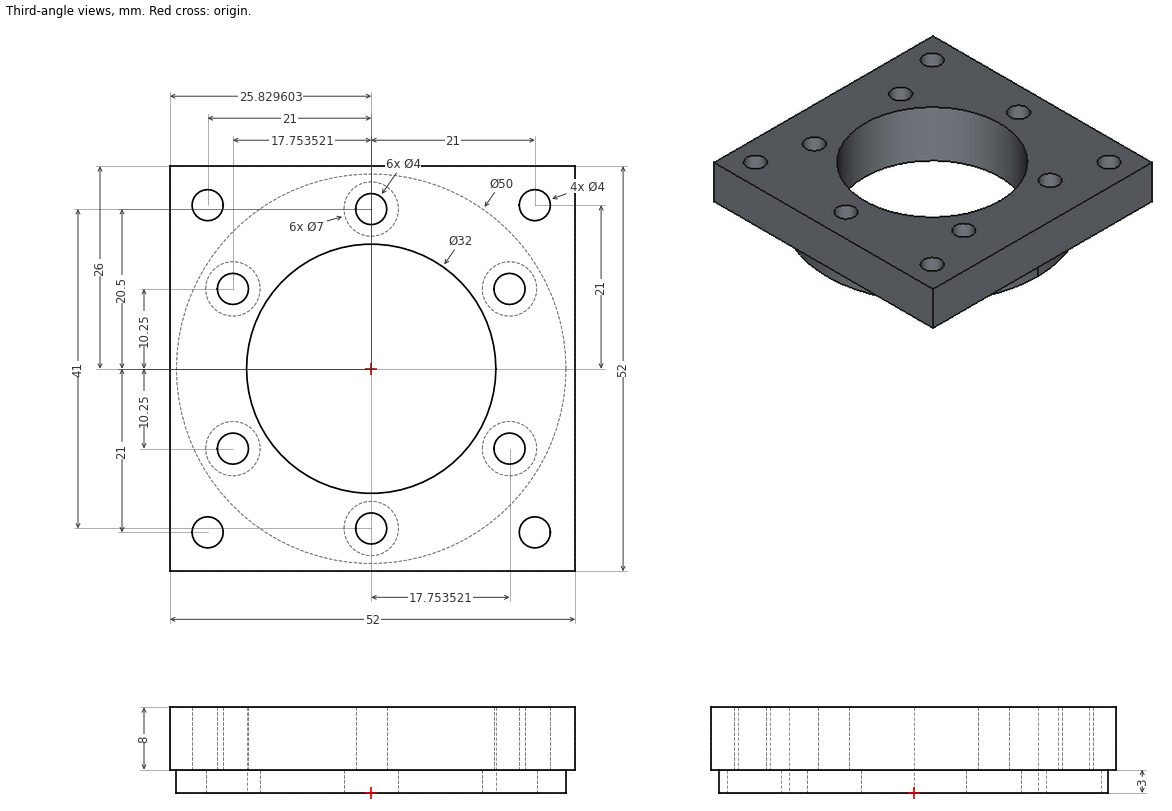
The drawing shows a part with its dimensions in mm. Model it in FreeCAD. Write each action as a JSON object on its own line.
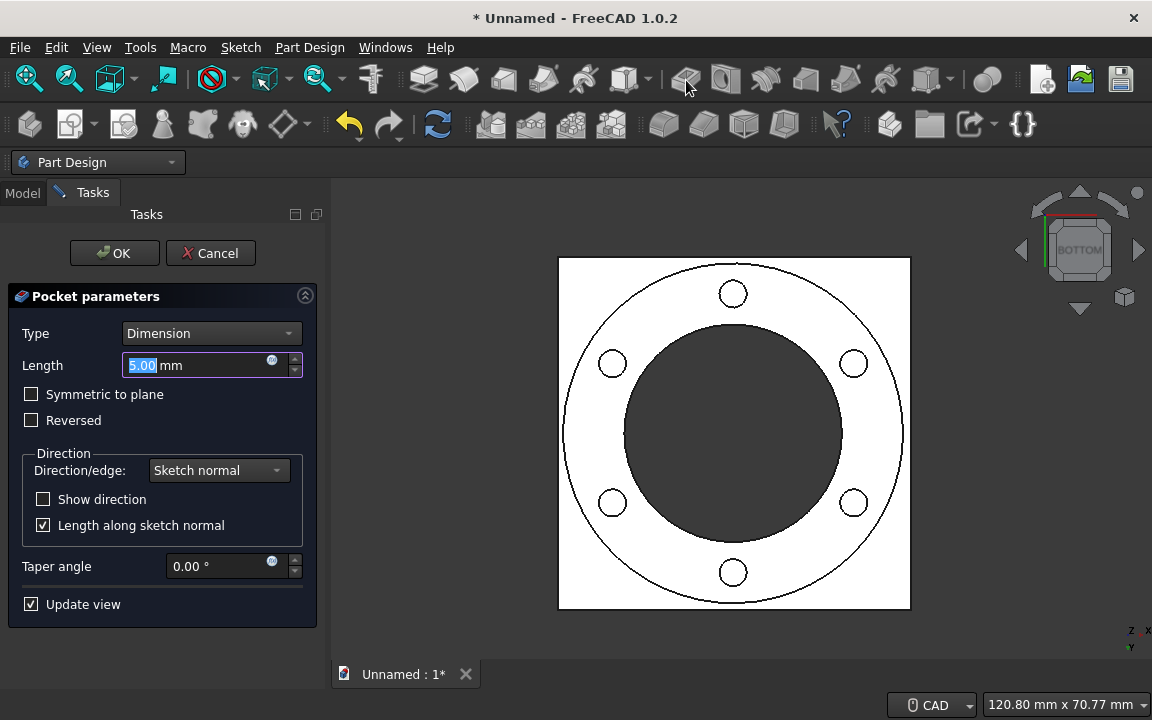
{"action": "left_click", "coordinate": [212, 334]}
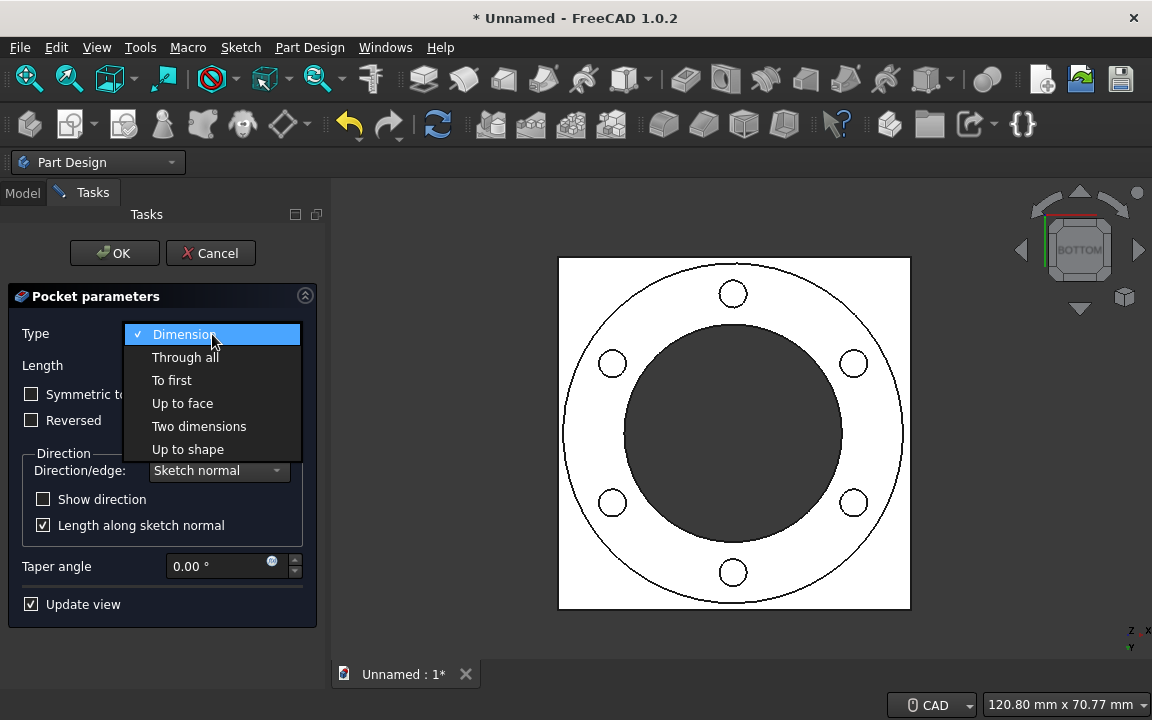
{"action": "left_click", "coordinate": [212, 358]}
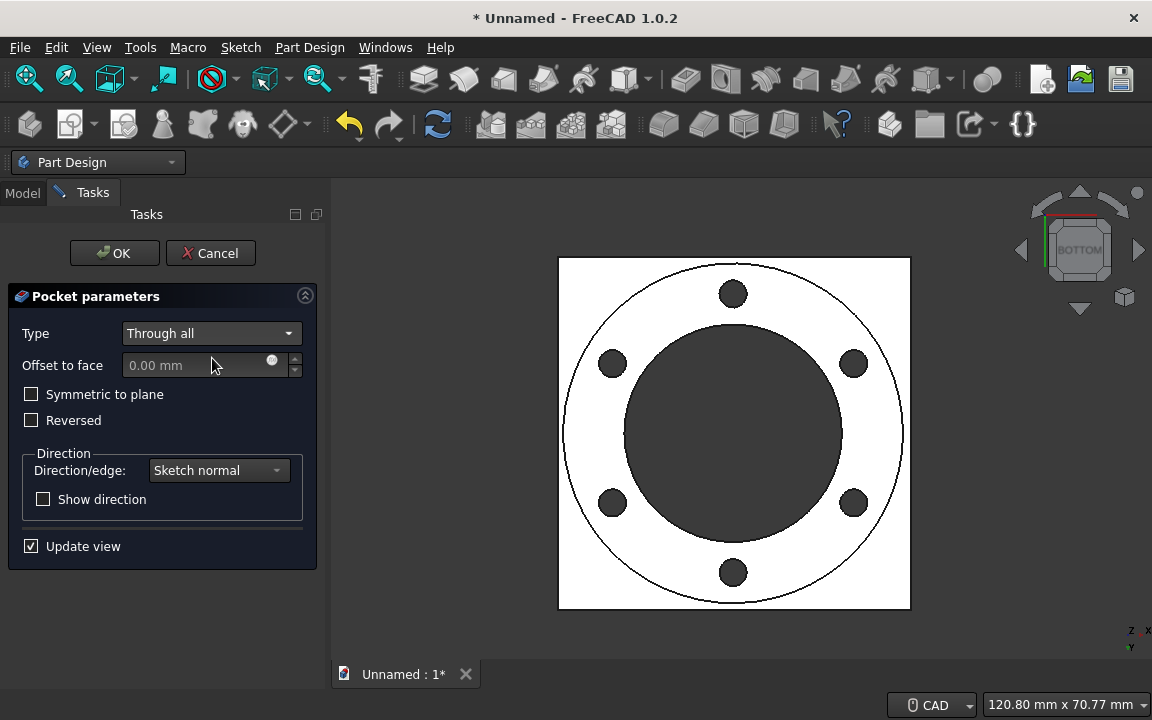
{"action": "left_click", "coordinate": [115, 253]}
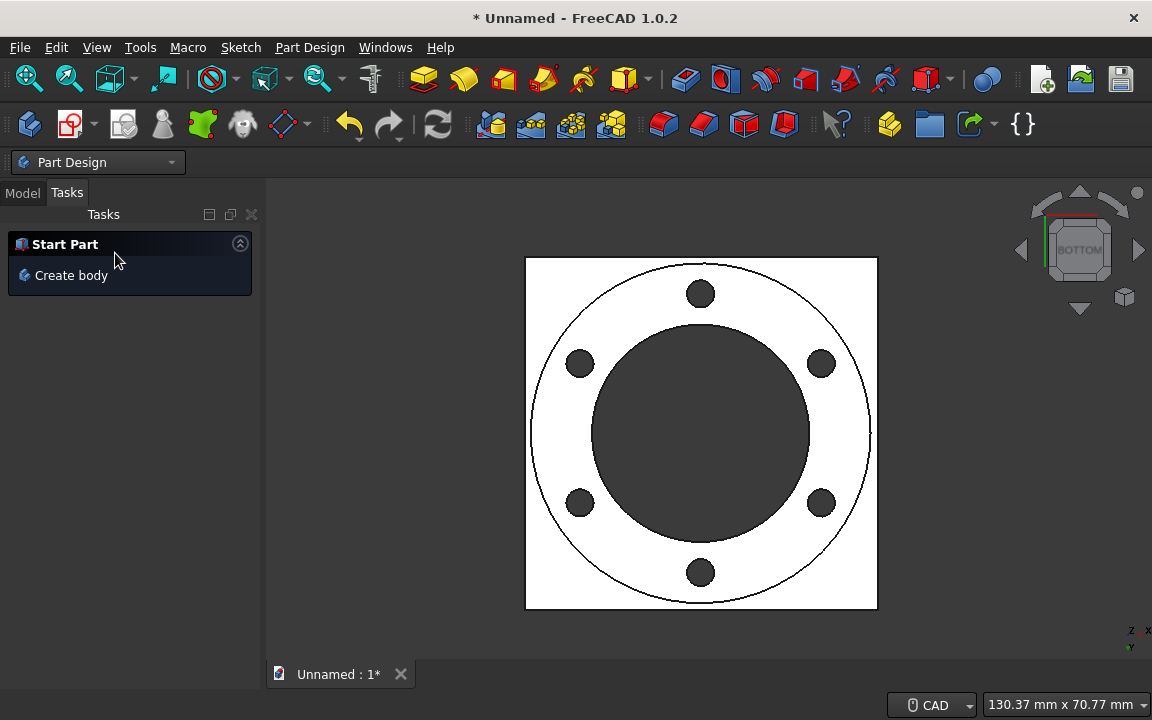
{"action": "left_click", "coordinate": [853, 584]}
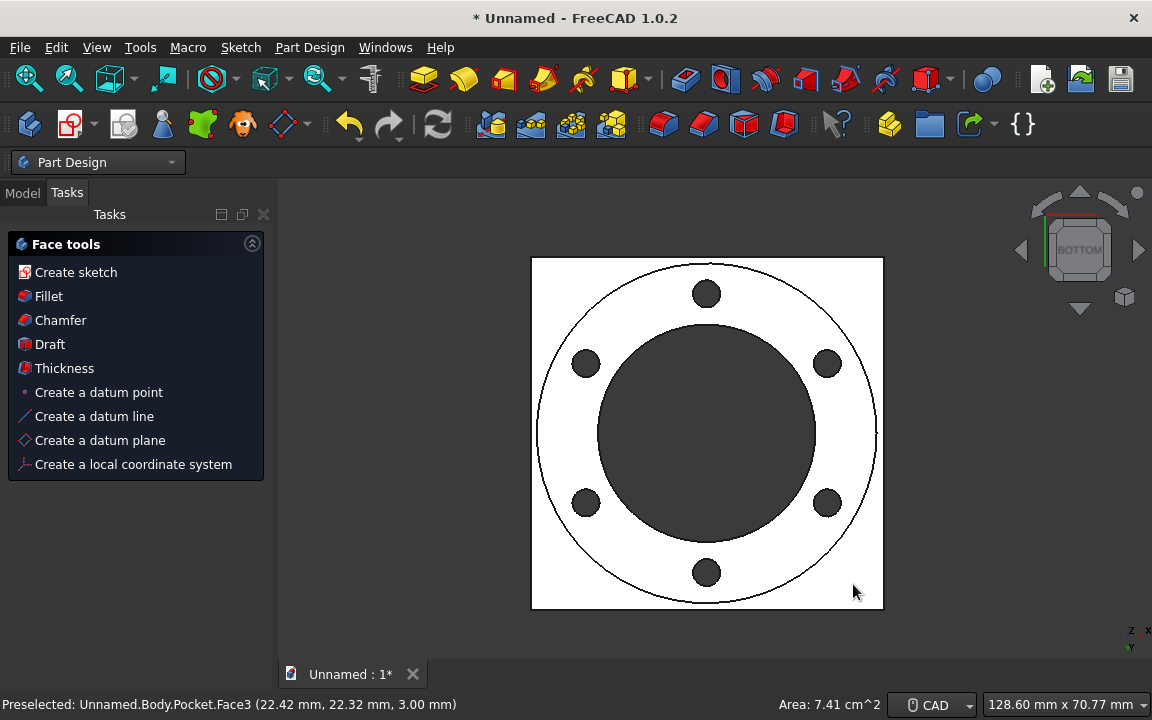
{"action": "left_click", "coordinate": [70, 124]}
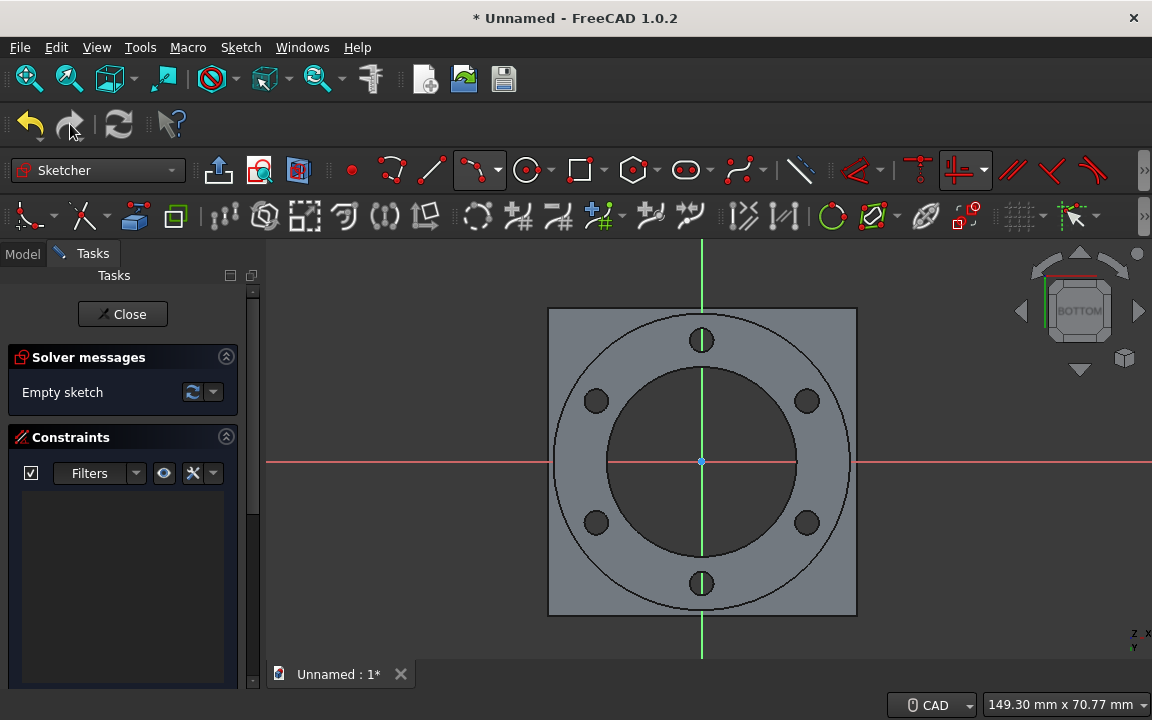
{"action": "left_click", "coordinate": [300, 170]}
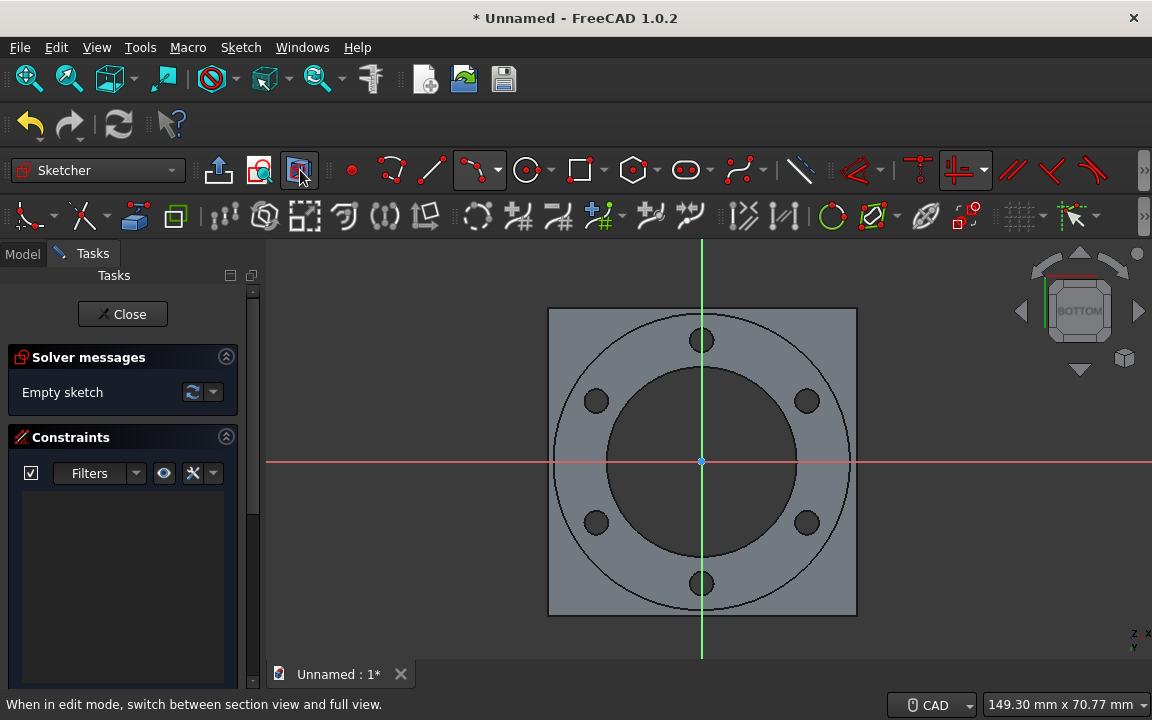
{"action": "key", "text": "g c"}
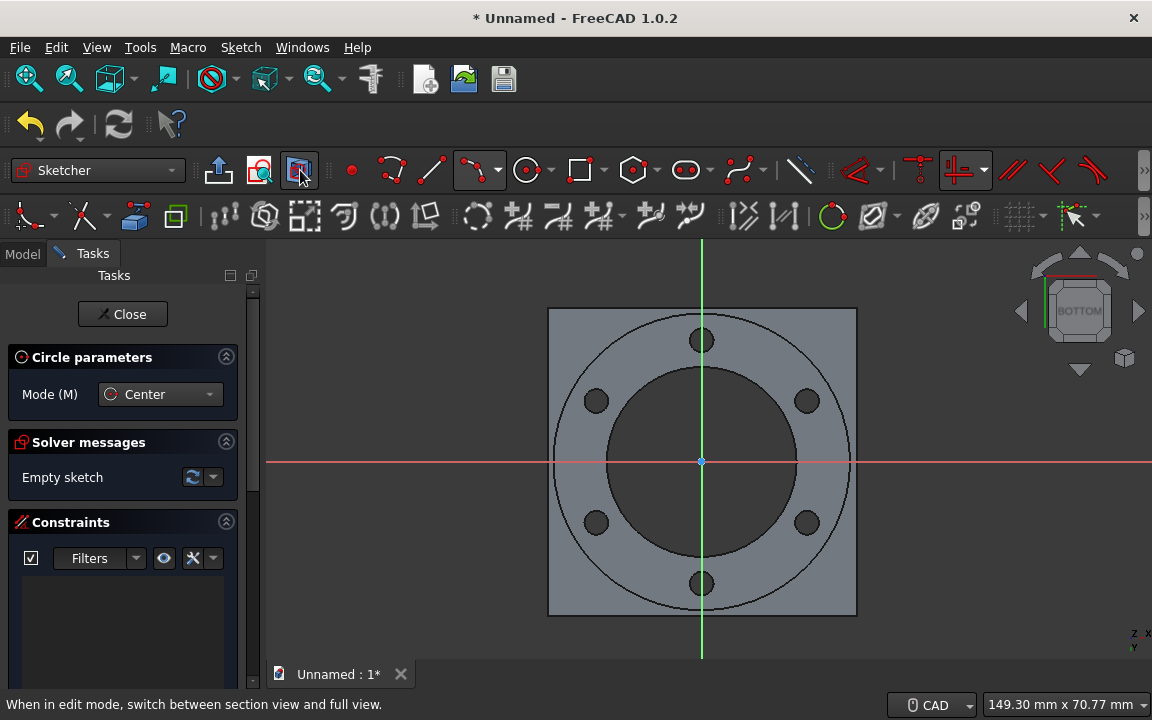
{"action": "scroll", "coordinate": [826, 587], "scroll_direction": "up", "scroll_amount": 4}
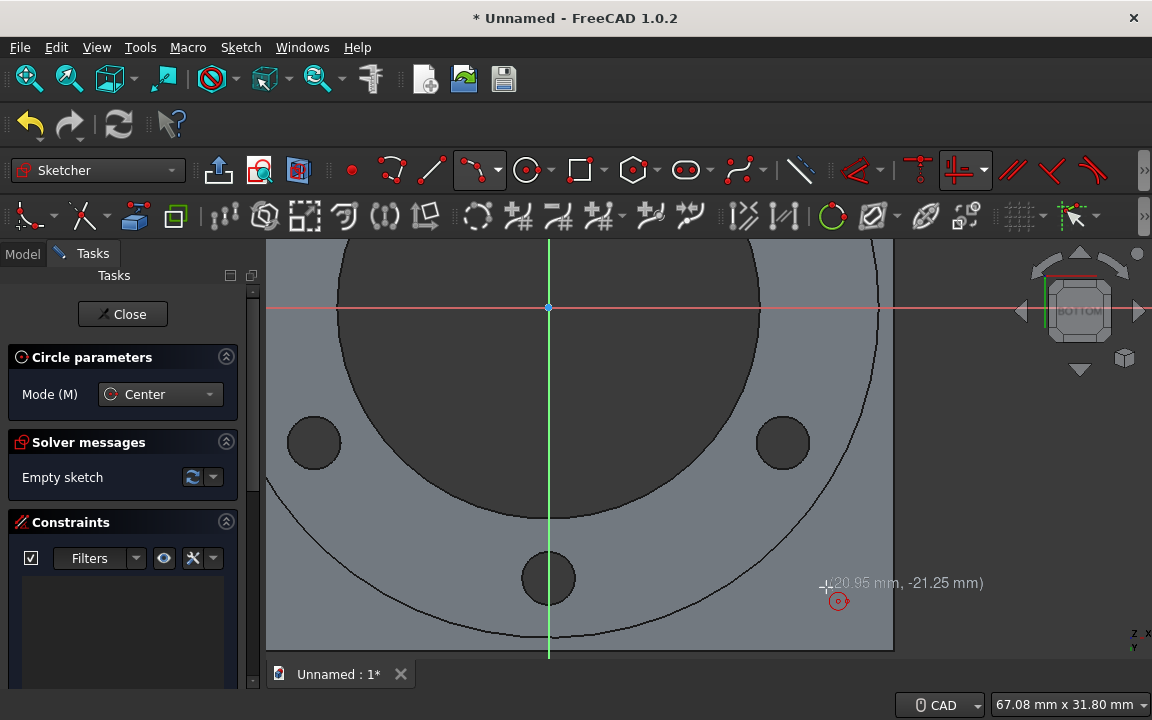
{"action": "left_click", "coordinate": [826, 585]}
{"action": "mouse_move", "coordinate": [845, 566]}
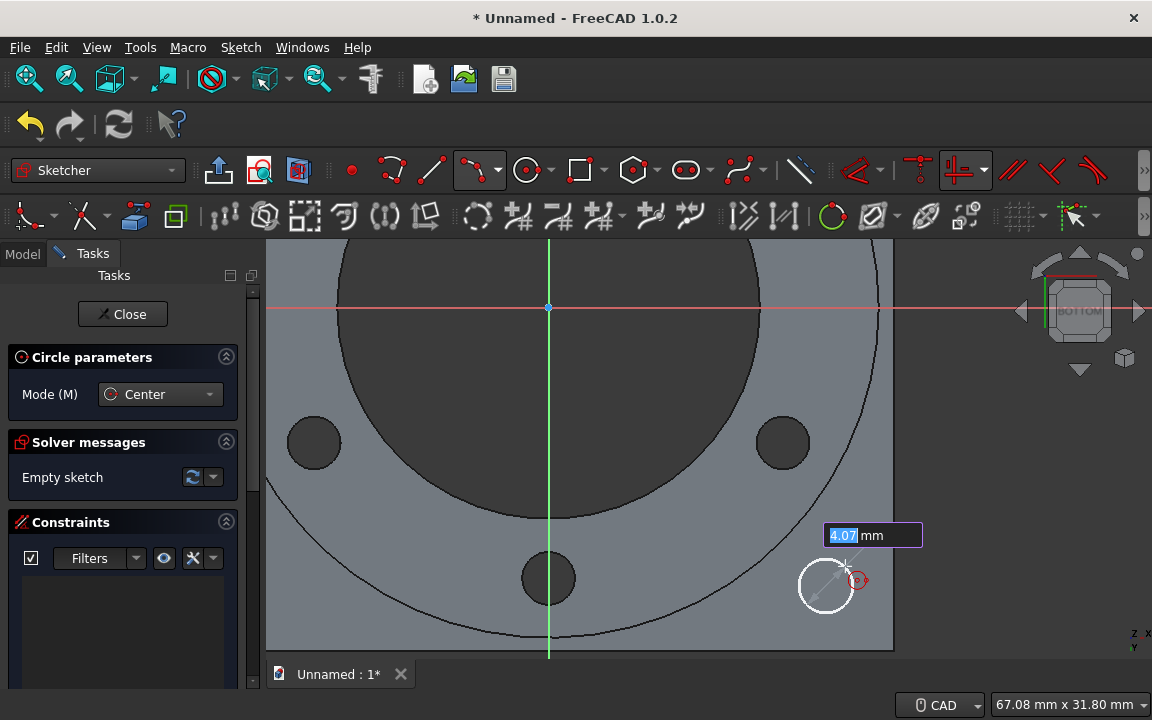
{"action": "type", "text": "4"}
{"action": "key", "text": "Return"}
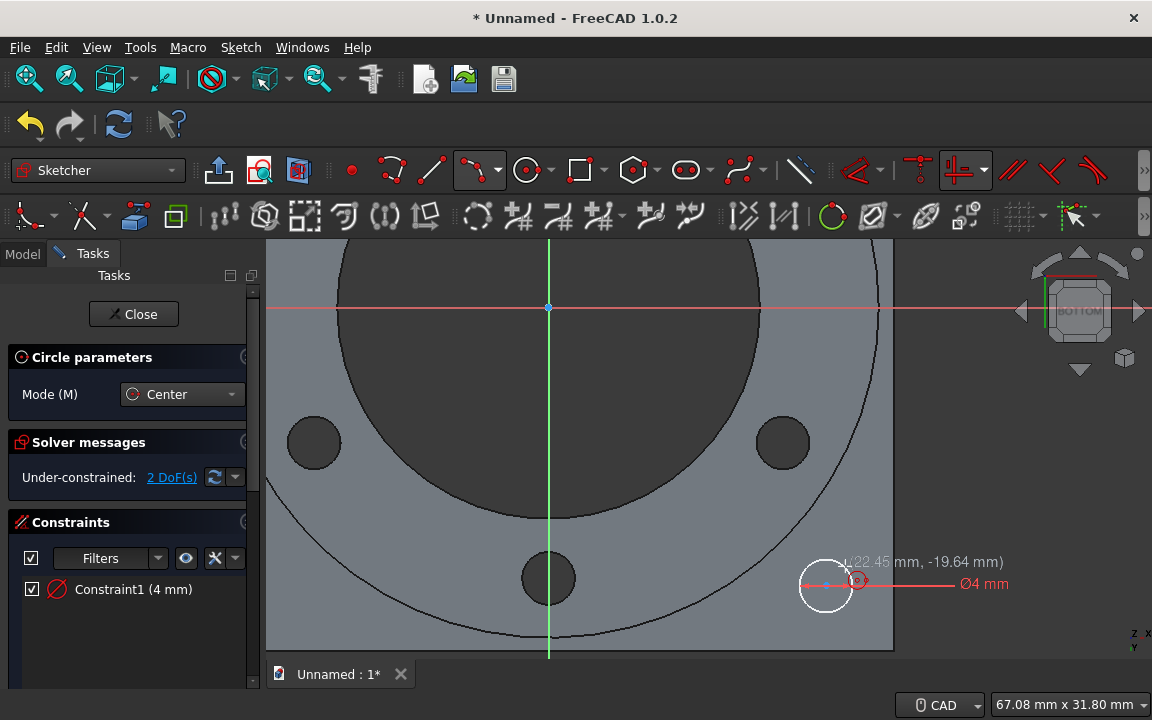
{"action": "scroll", "coordinate": [716, 564], "scroll_direction": "down", "scroll_amount": 4}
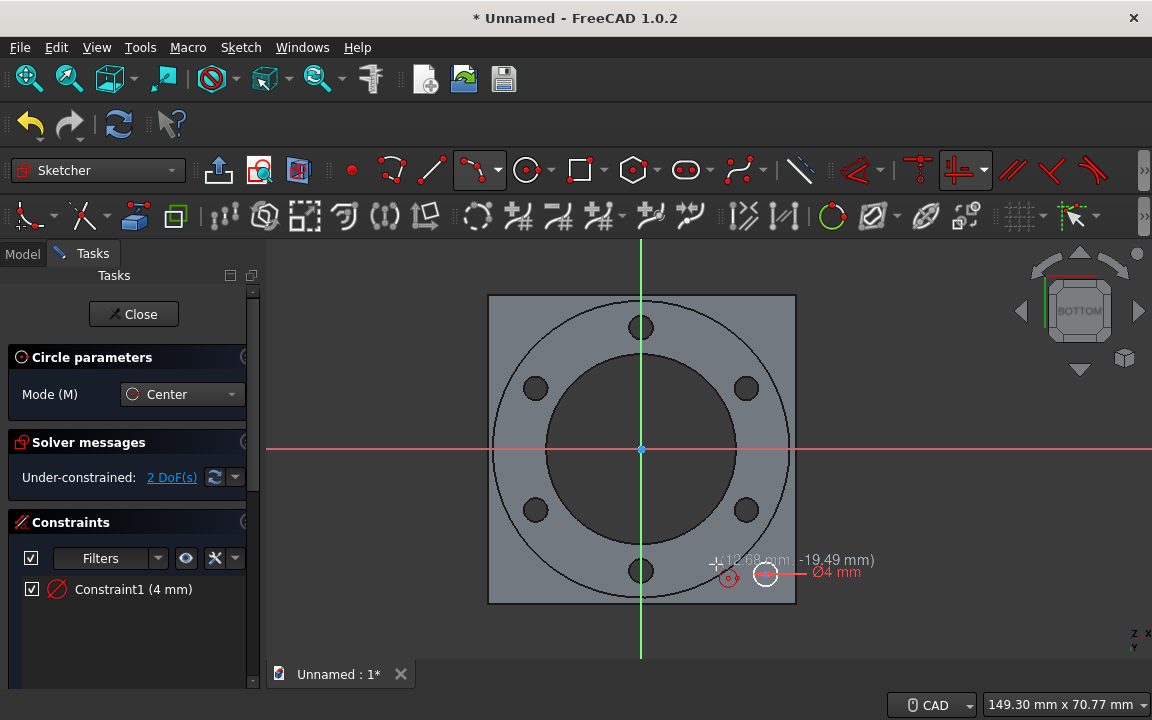
{"action": "scroll", "coordinate": [516, 574], "scroll_direction": "up", "scroll_amount": 4}